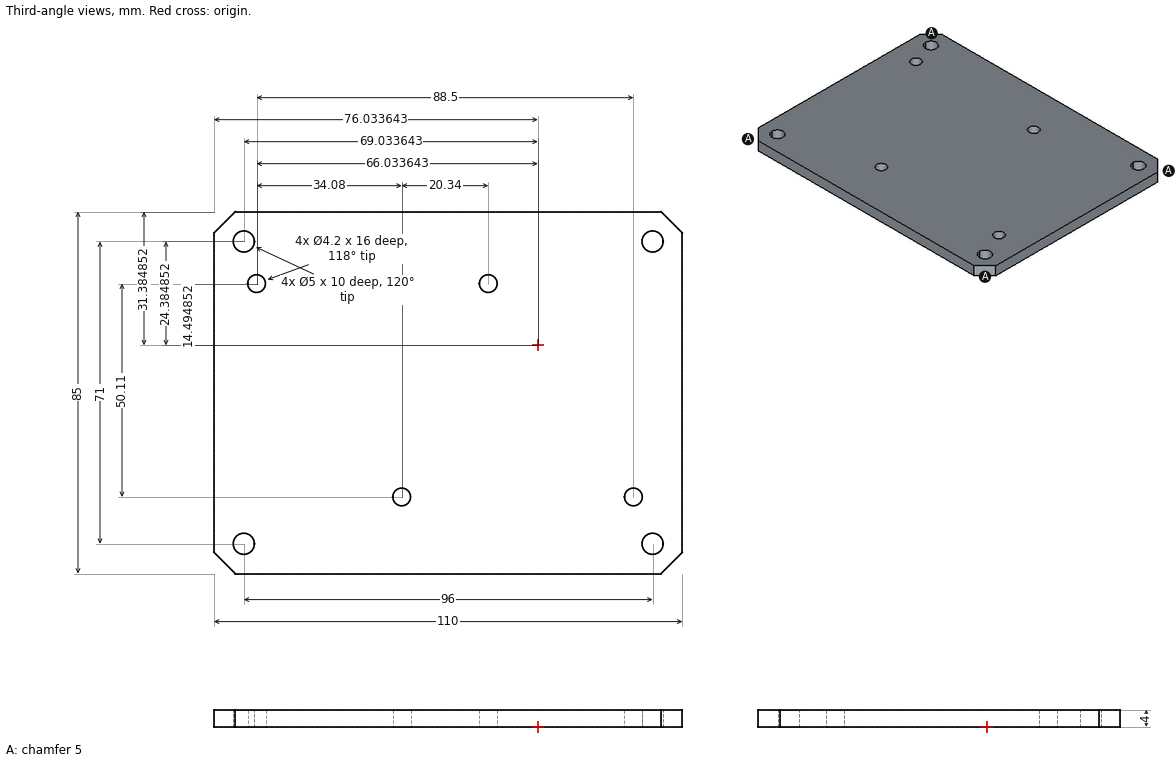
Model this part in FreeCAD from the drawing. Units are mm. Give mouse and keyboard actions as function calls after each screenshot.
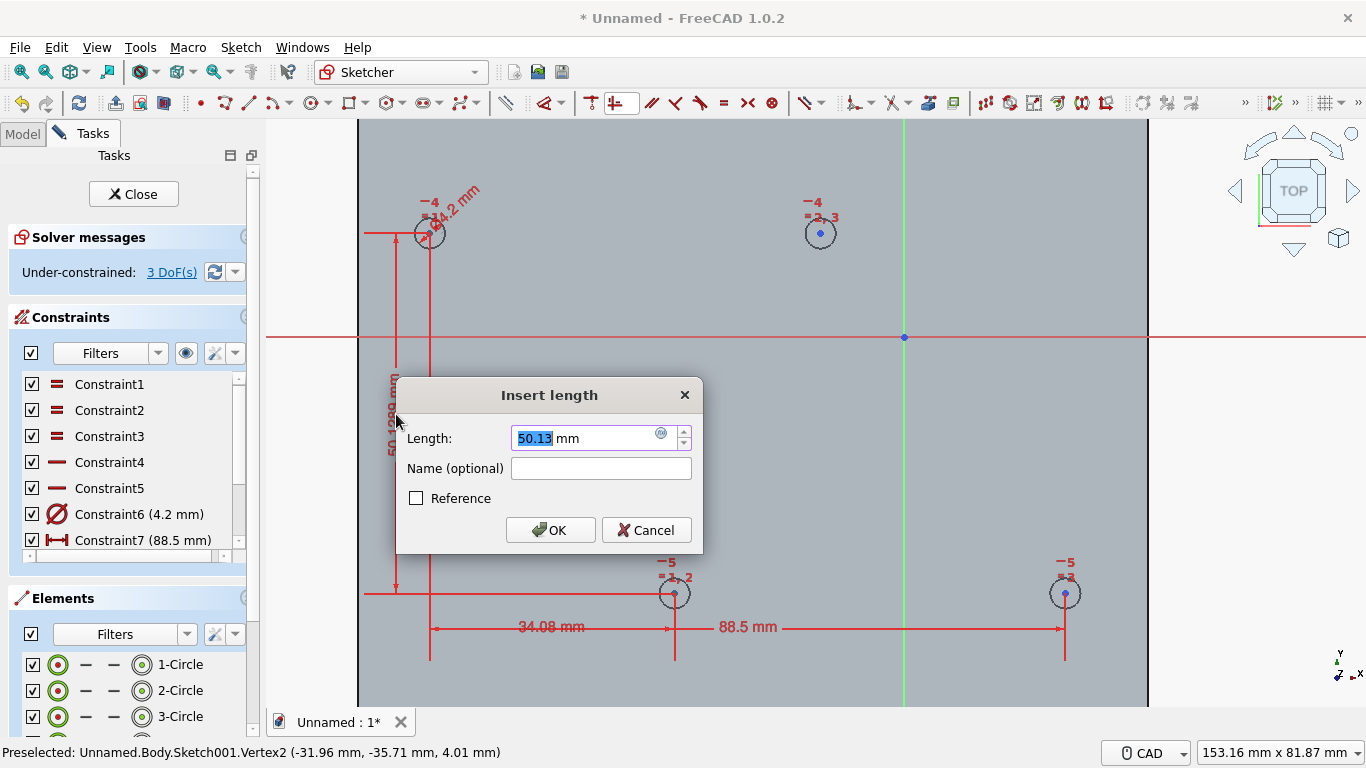
text(50.11)
key(Return)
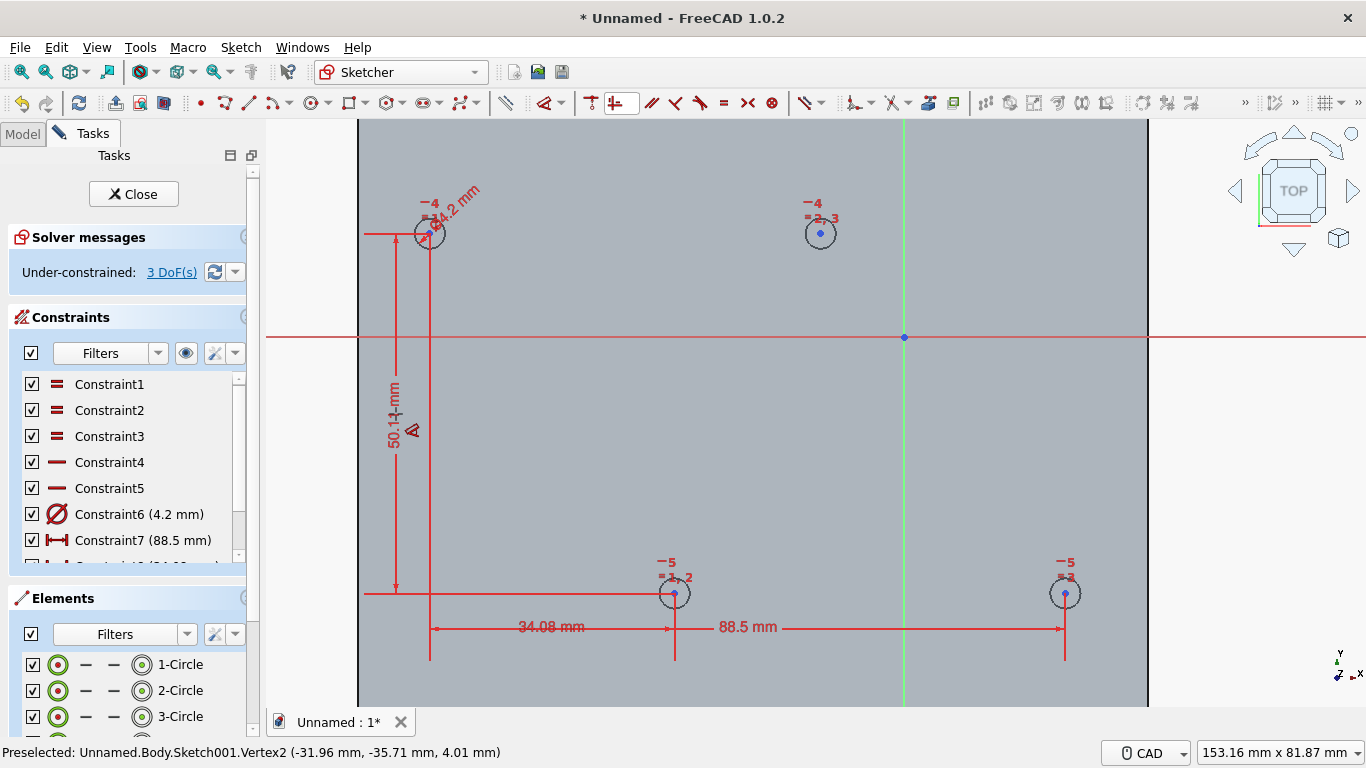
click(675, 594)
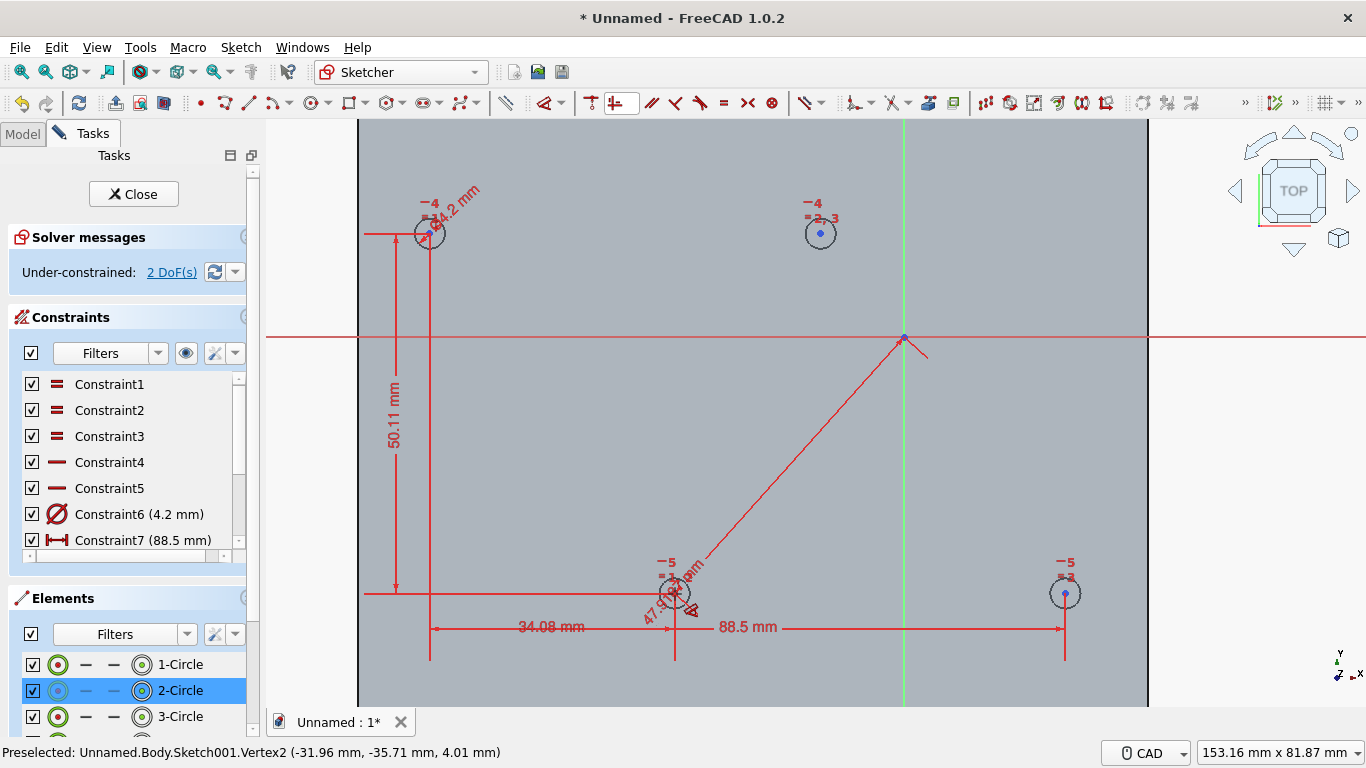
click(821, 234)
click(748, 200)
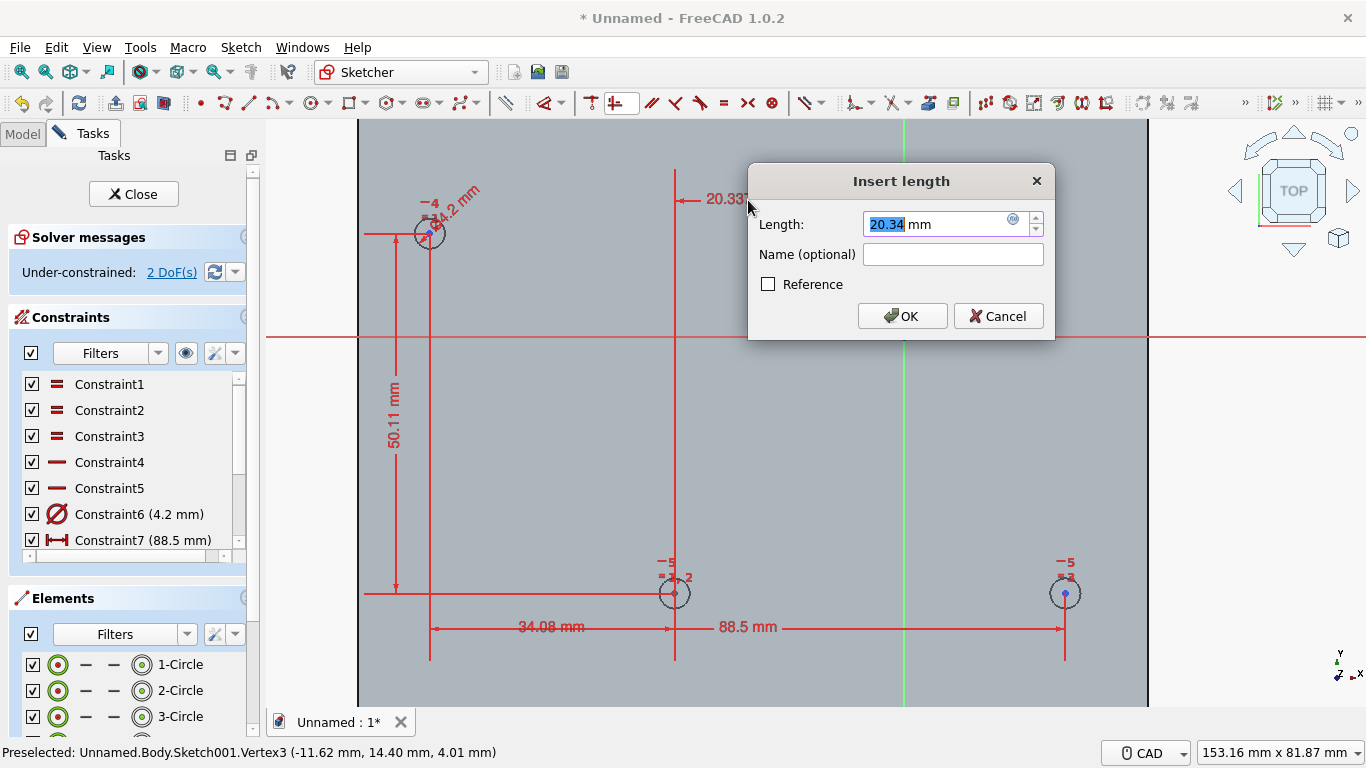
text(20.34)
key(Return)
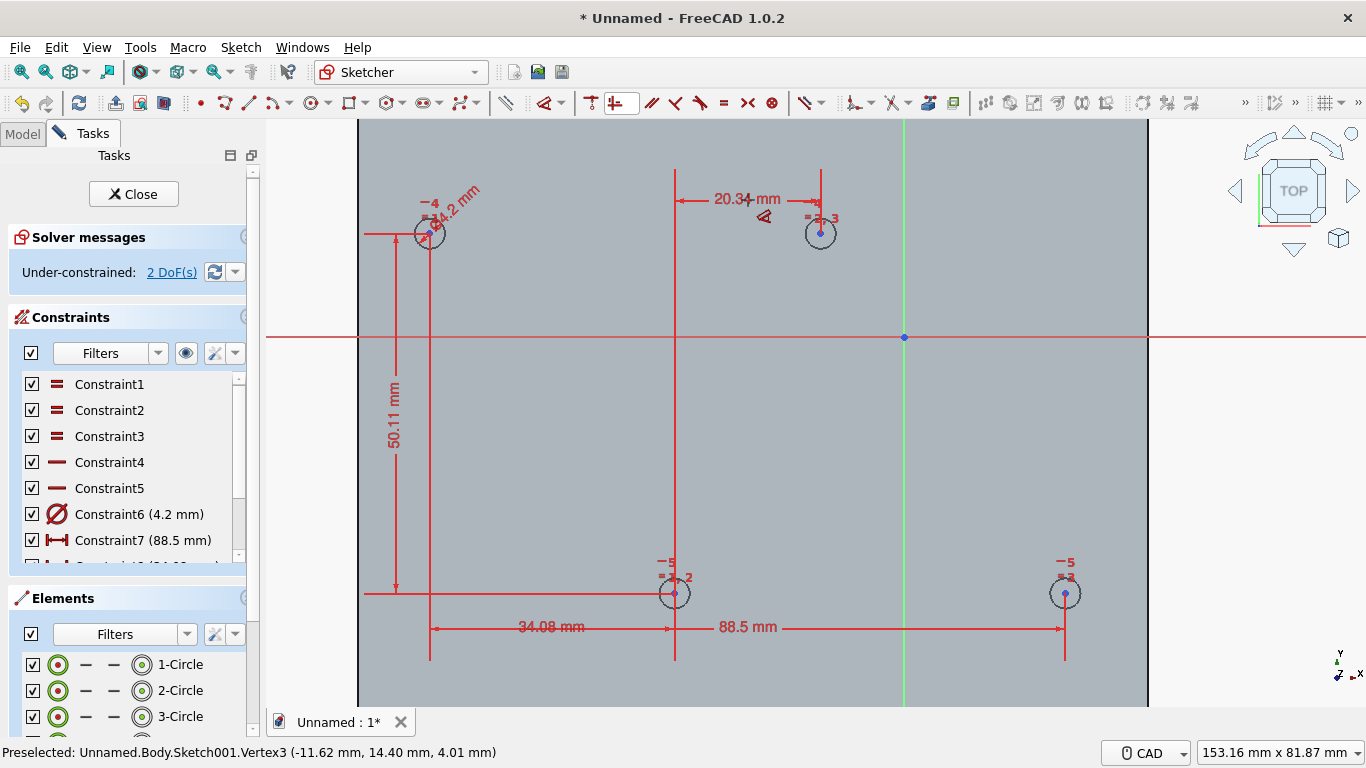
click(430, 234)
click(667, 200)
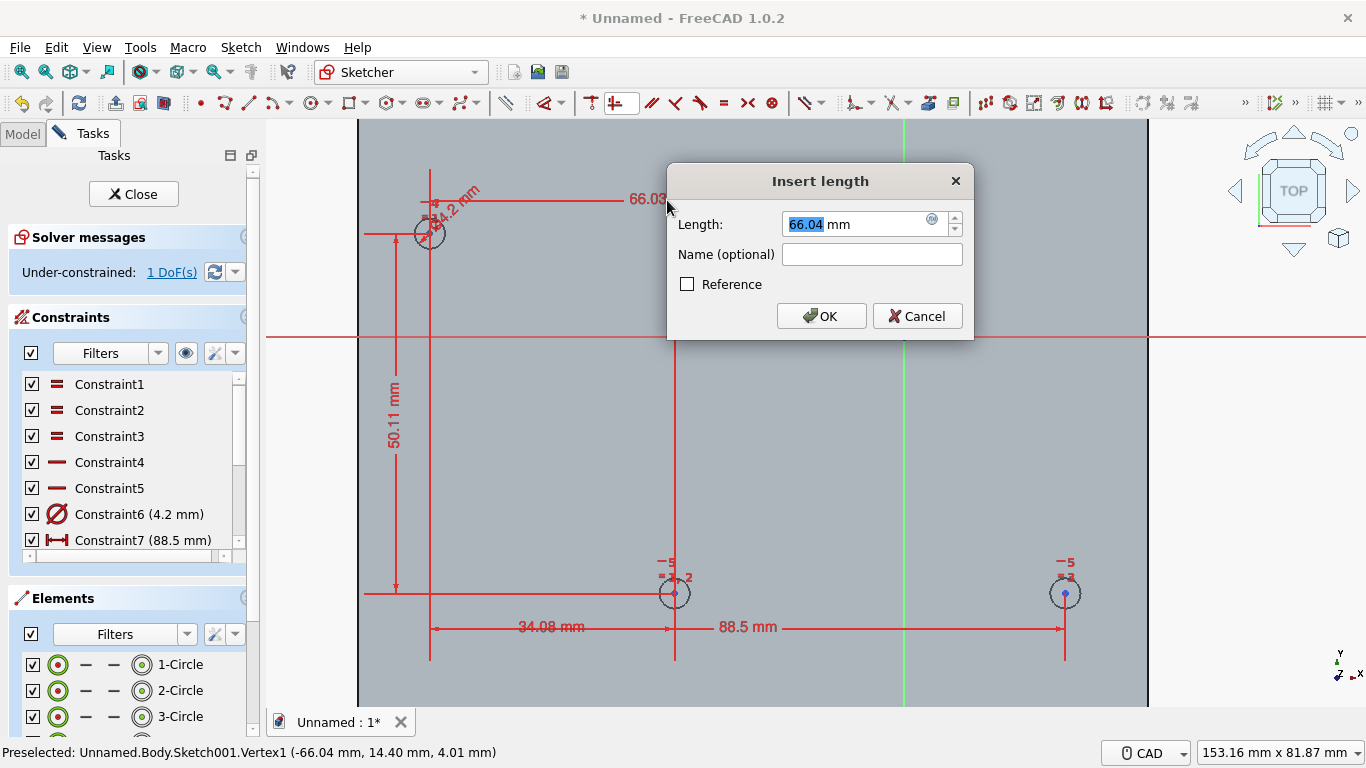
text(66.033643)
key(Return)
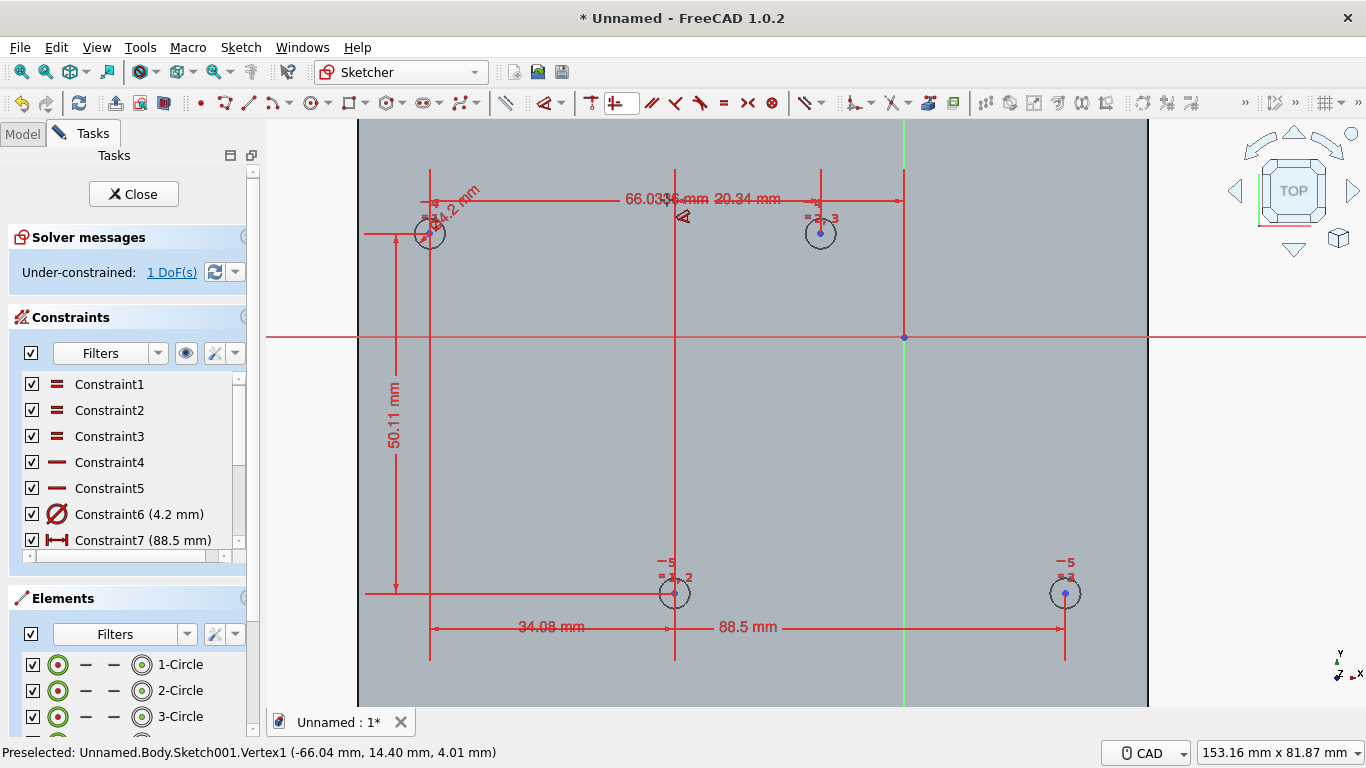
click(430, 234)
click(396, 285)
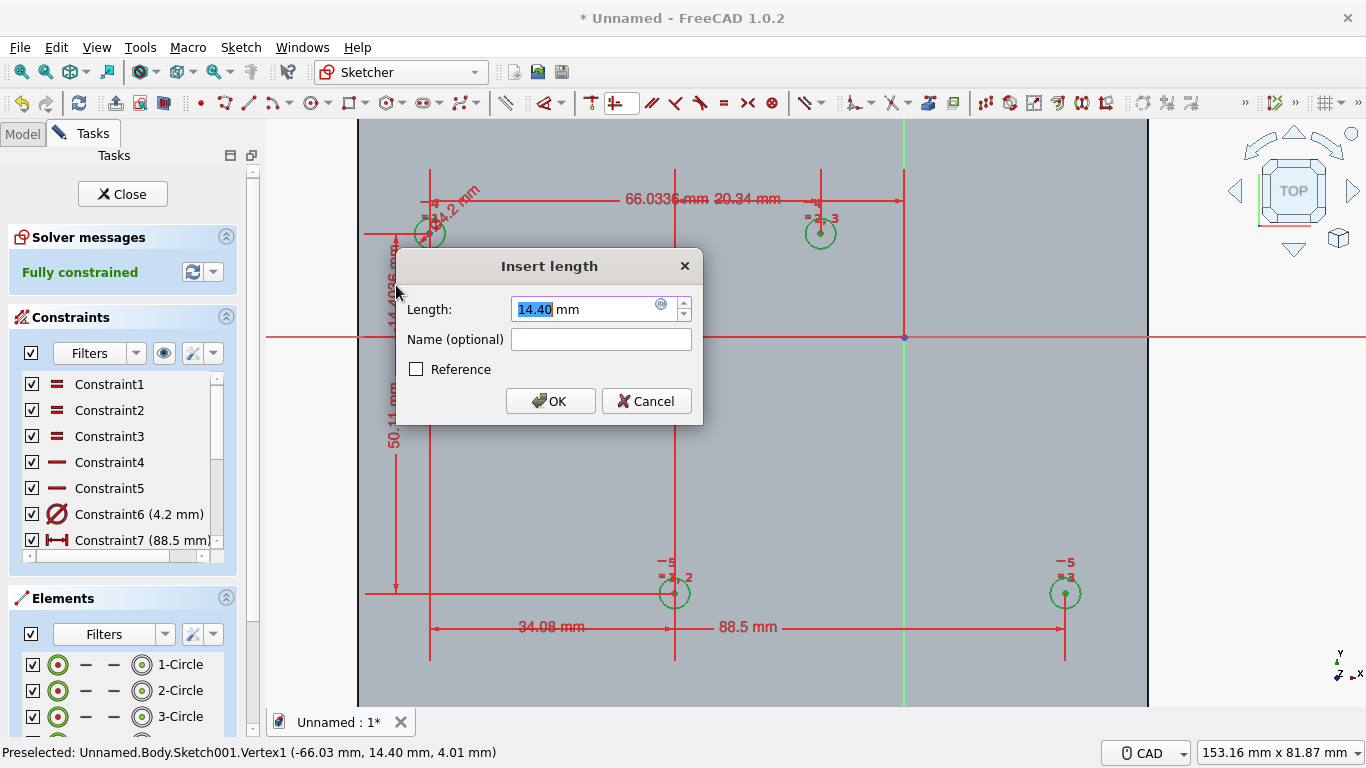
text(14.494852)
key(Return)
key(Escape)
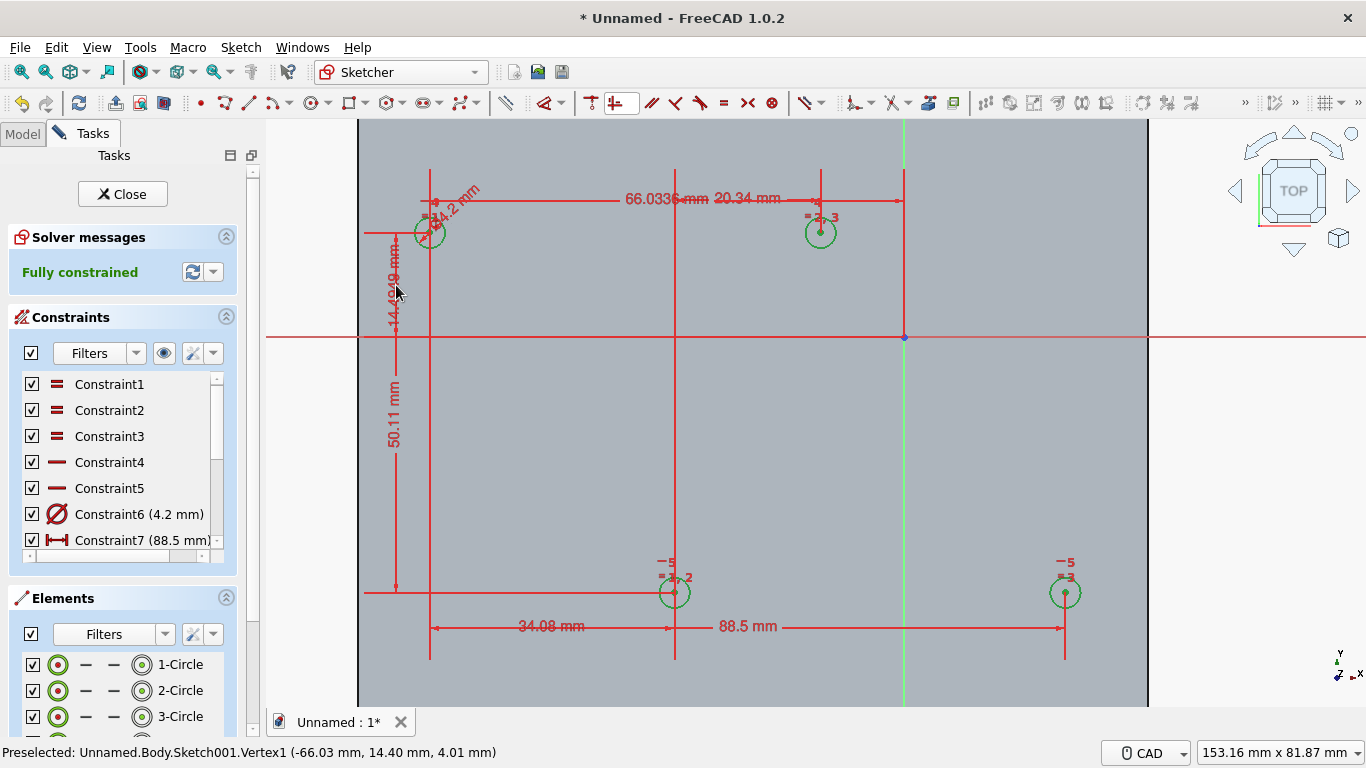
click(123, 194)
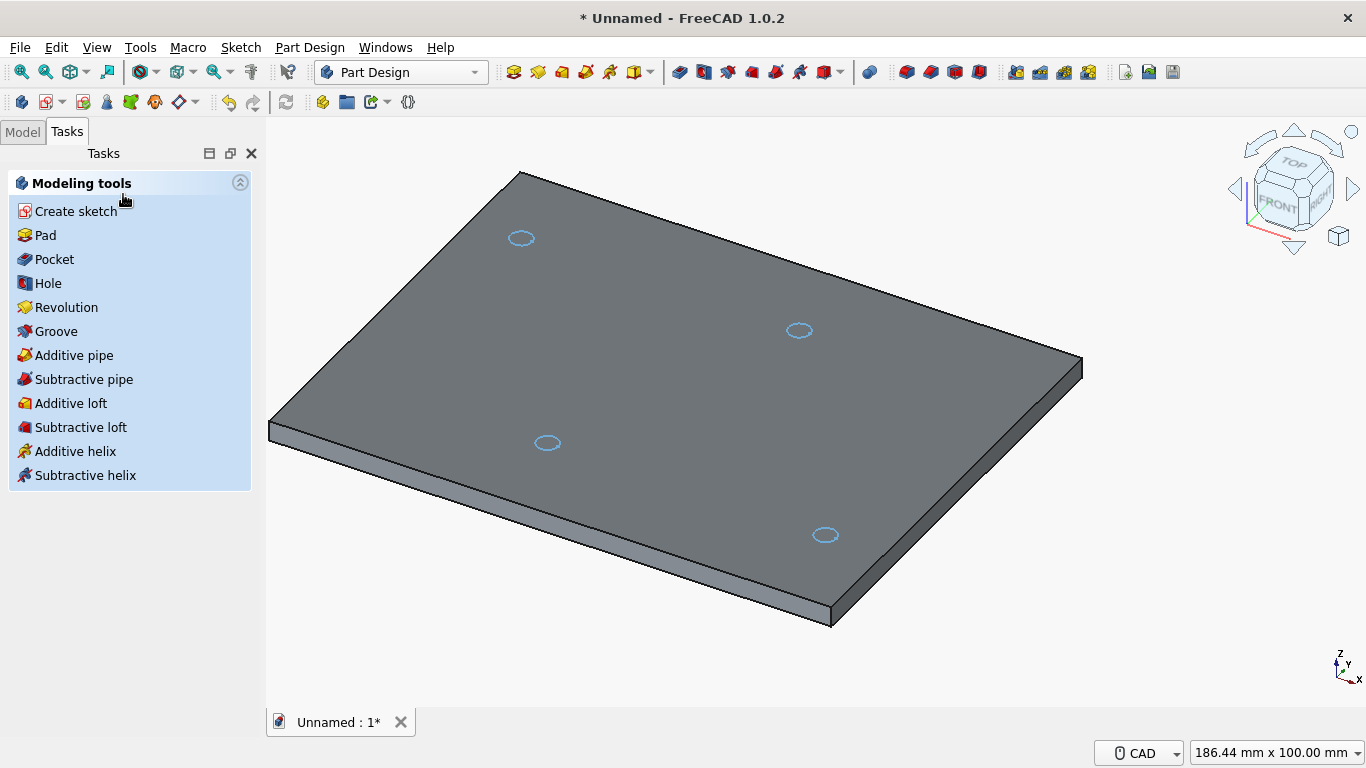
click(704, 72)